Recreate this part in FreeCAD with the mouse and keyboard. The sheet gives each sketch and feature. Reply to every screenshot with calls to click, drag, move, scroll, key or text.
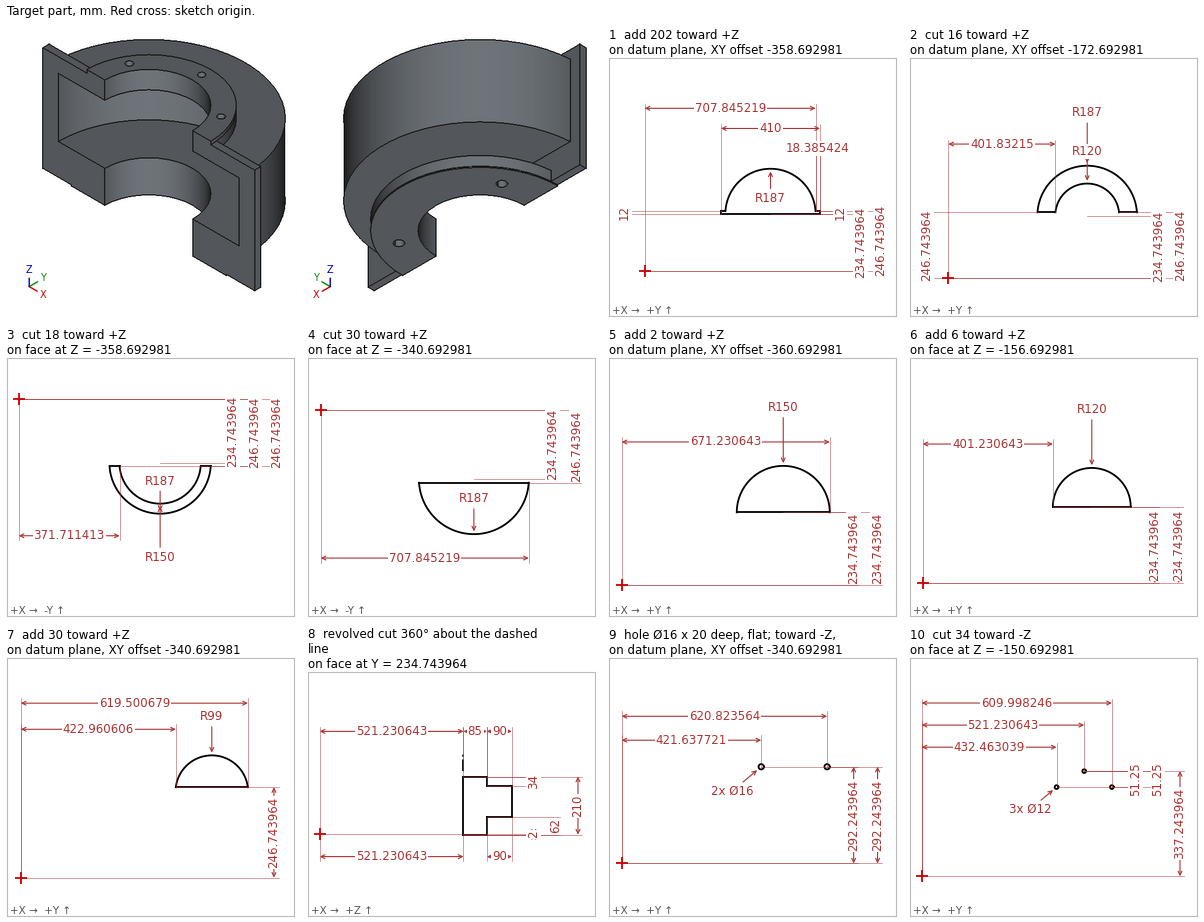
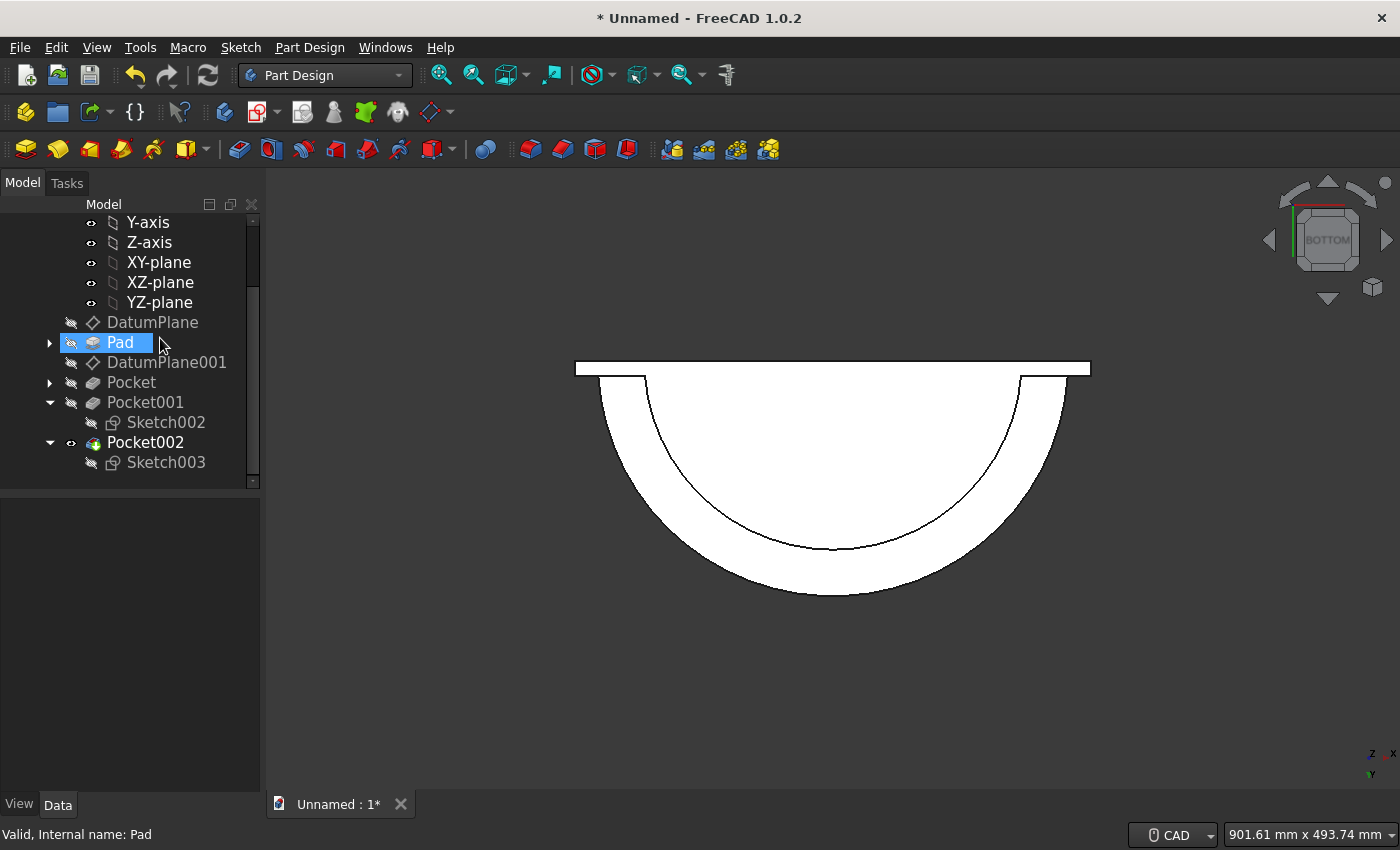
scroll(160, 338, up, 15)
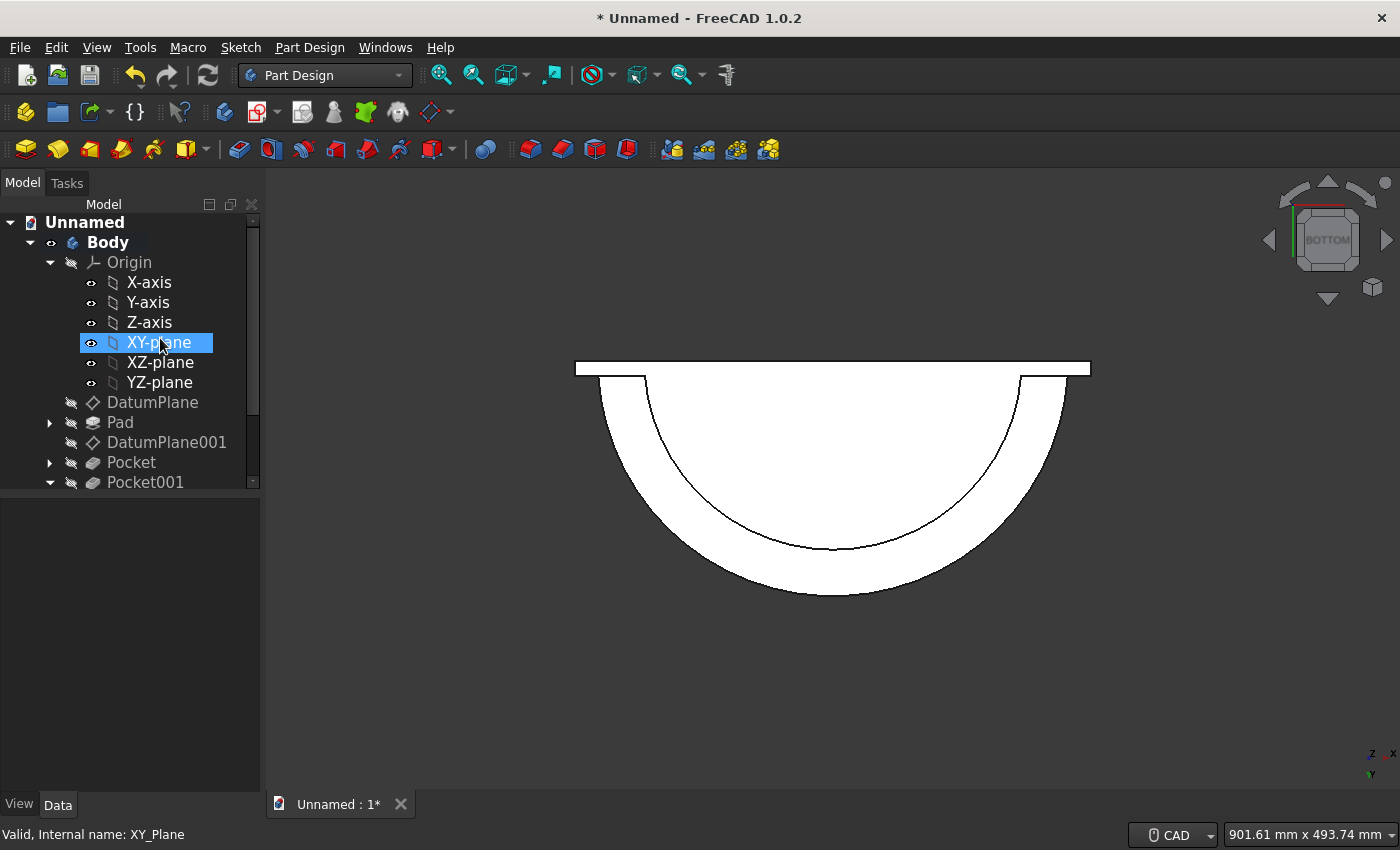
click(136, 343)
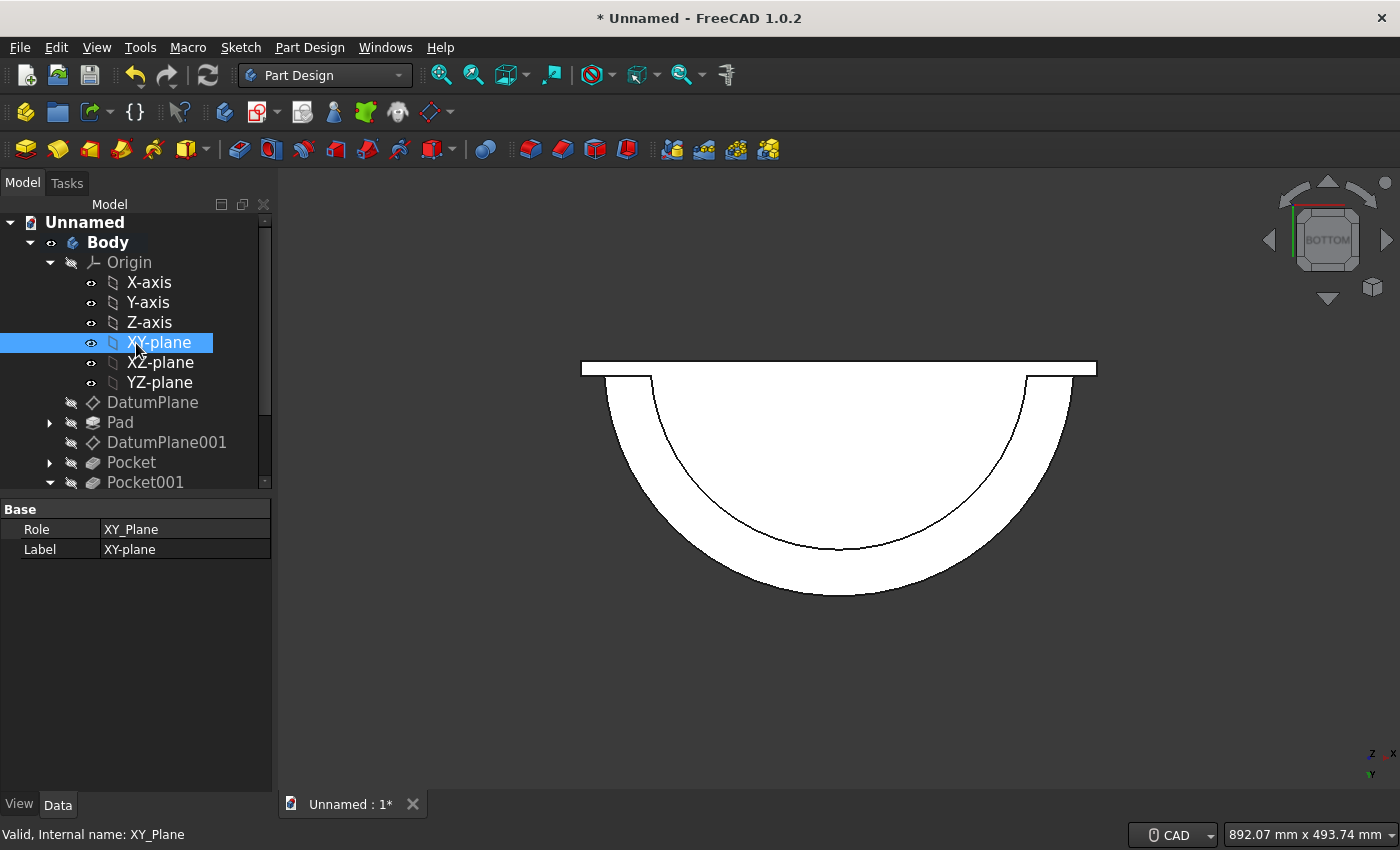
click(430, 112)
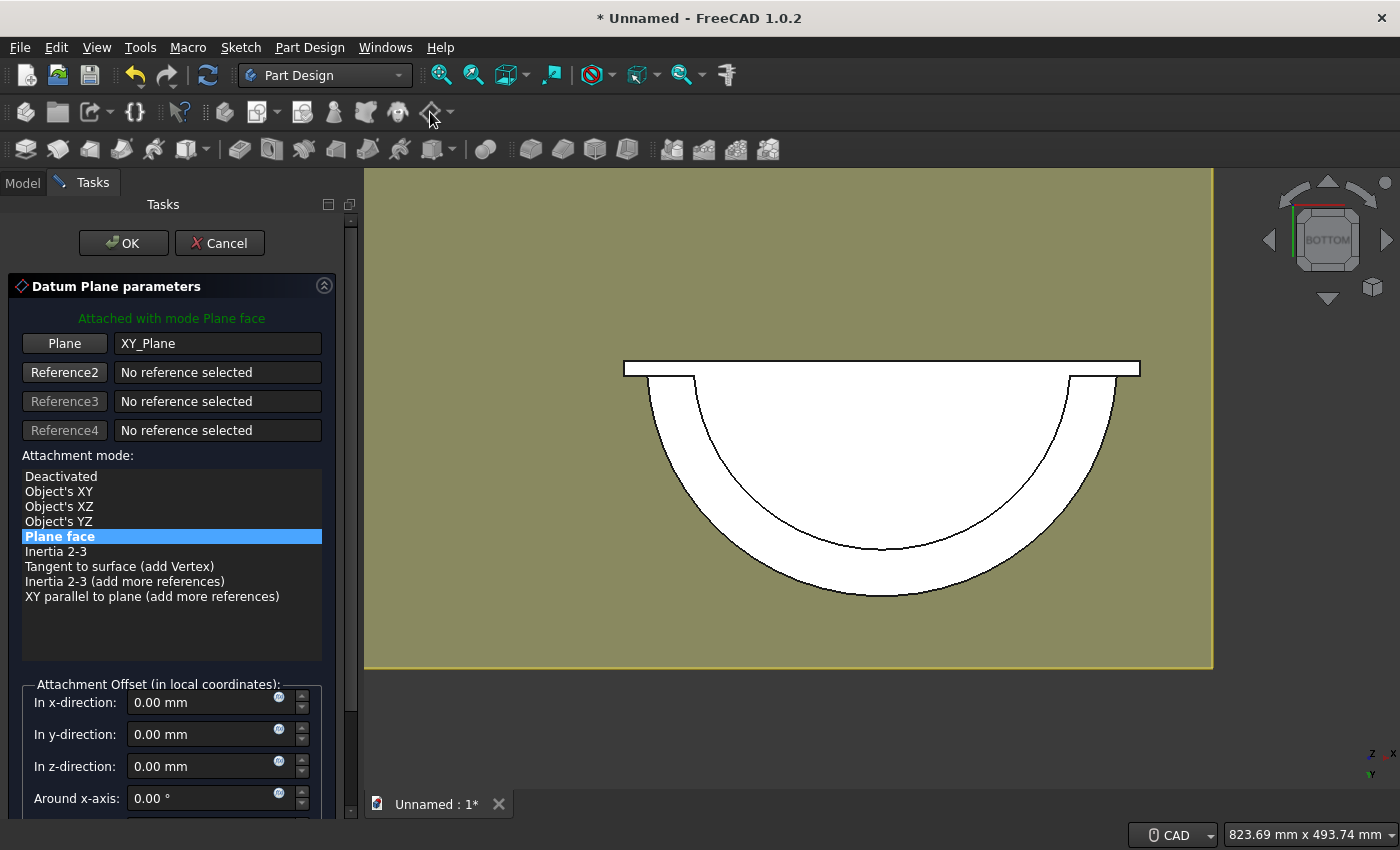
triple_click(210, 766)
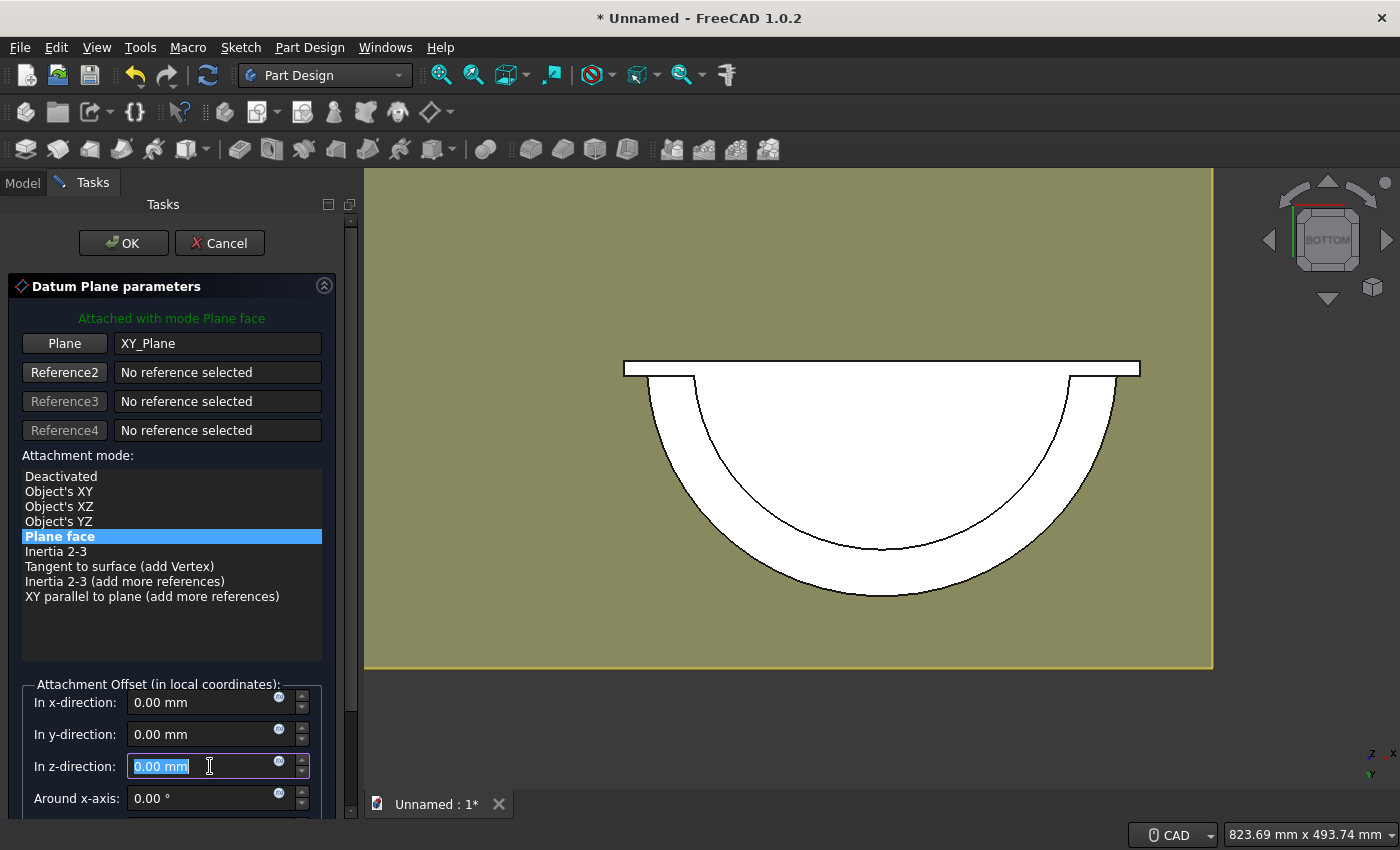
text(-360.692981)
key(Tab)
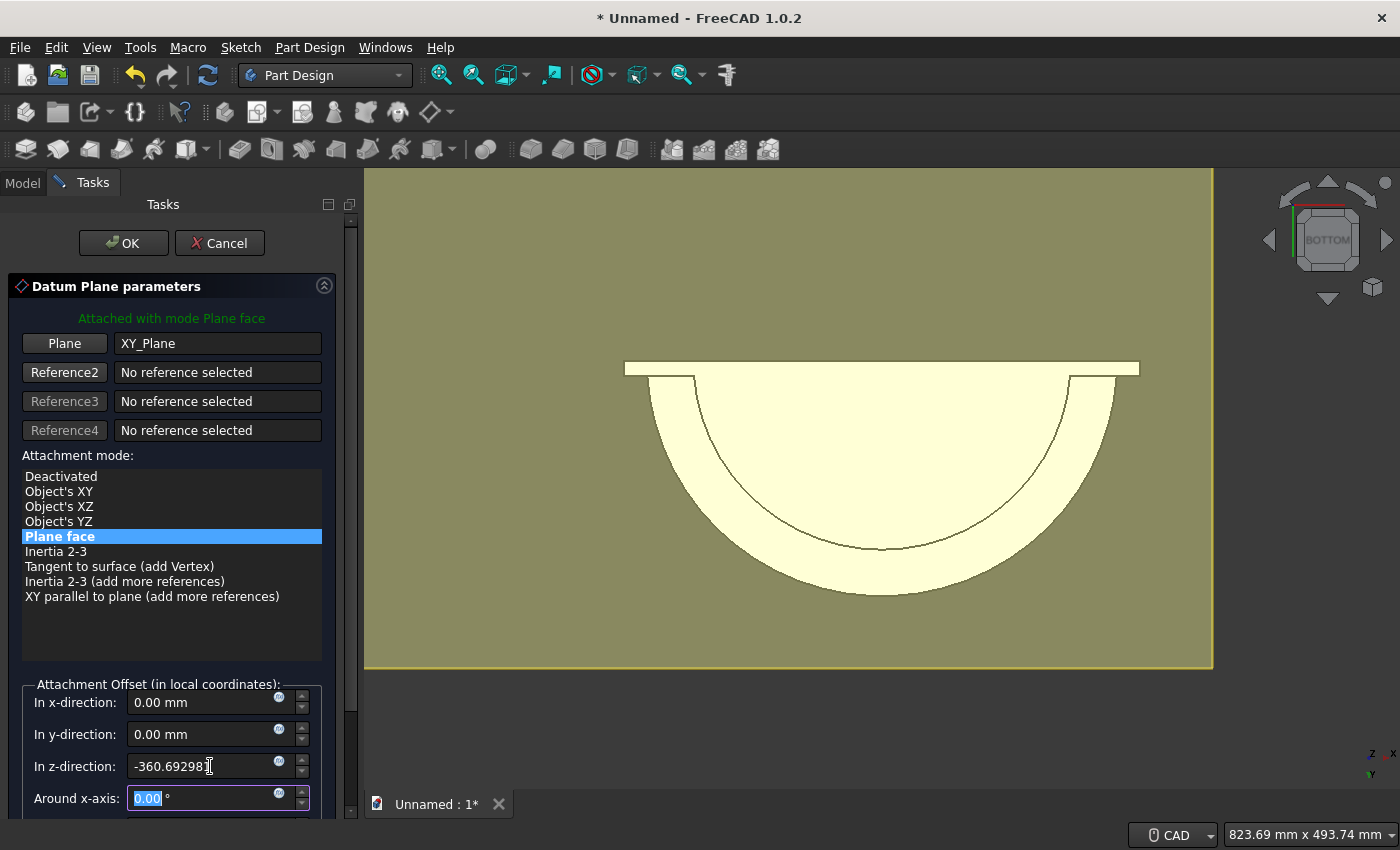
click(124, 243)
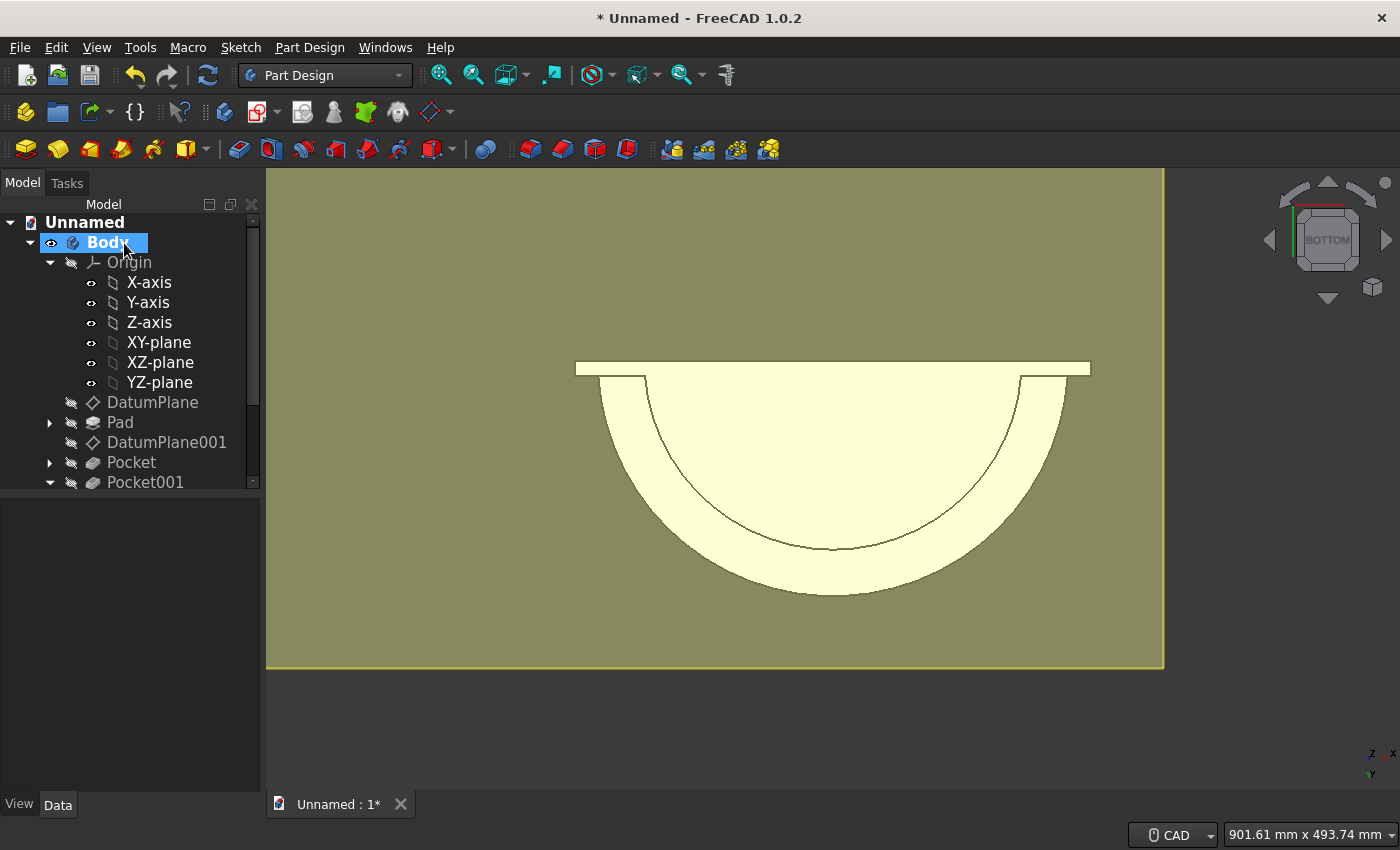
scroll(100, 358, down, 3)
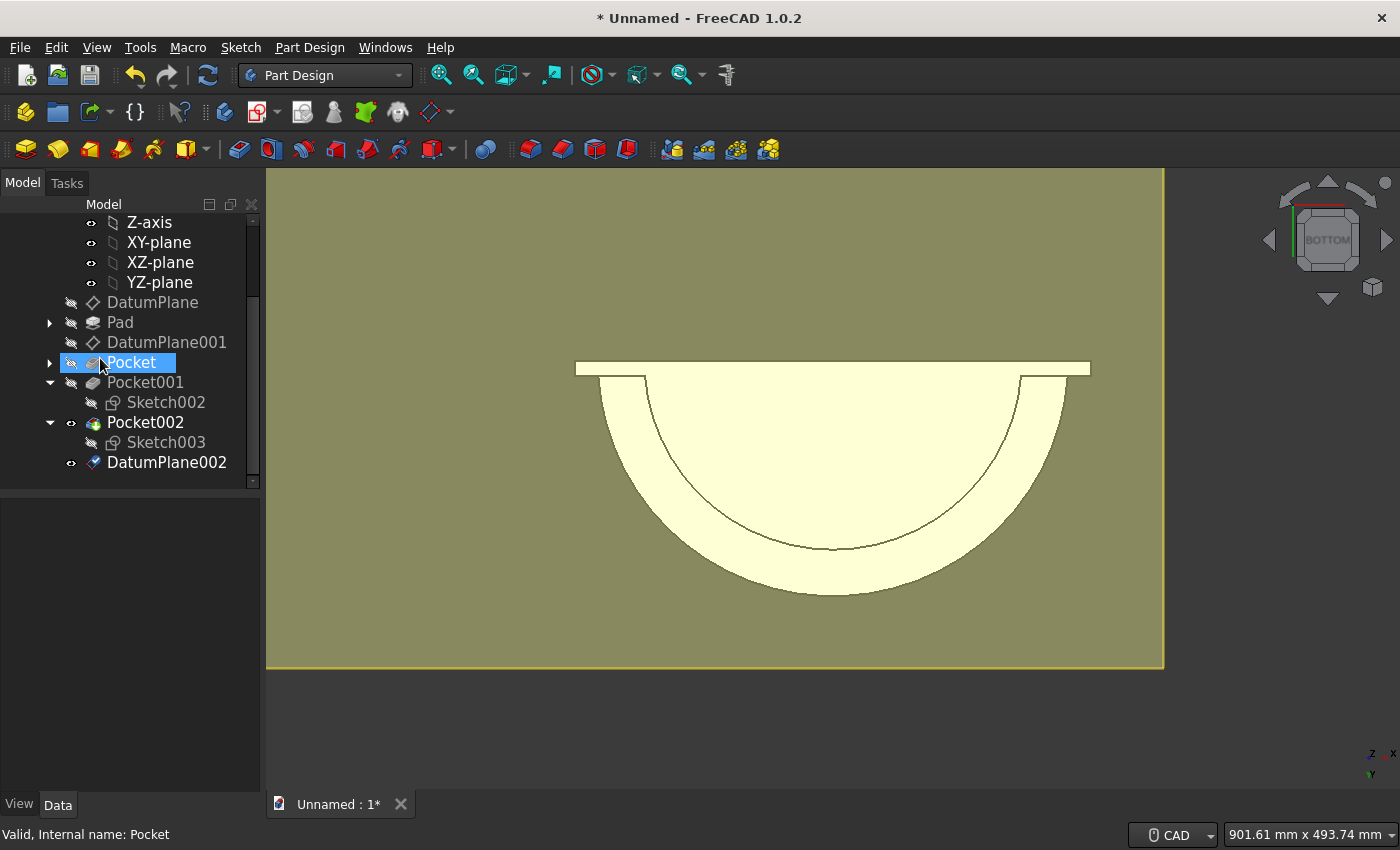
click(116, 463)